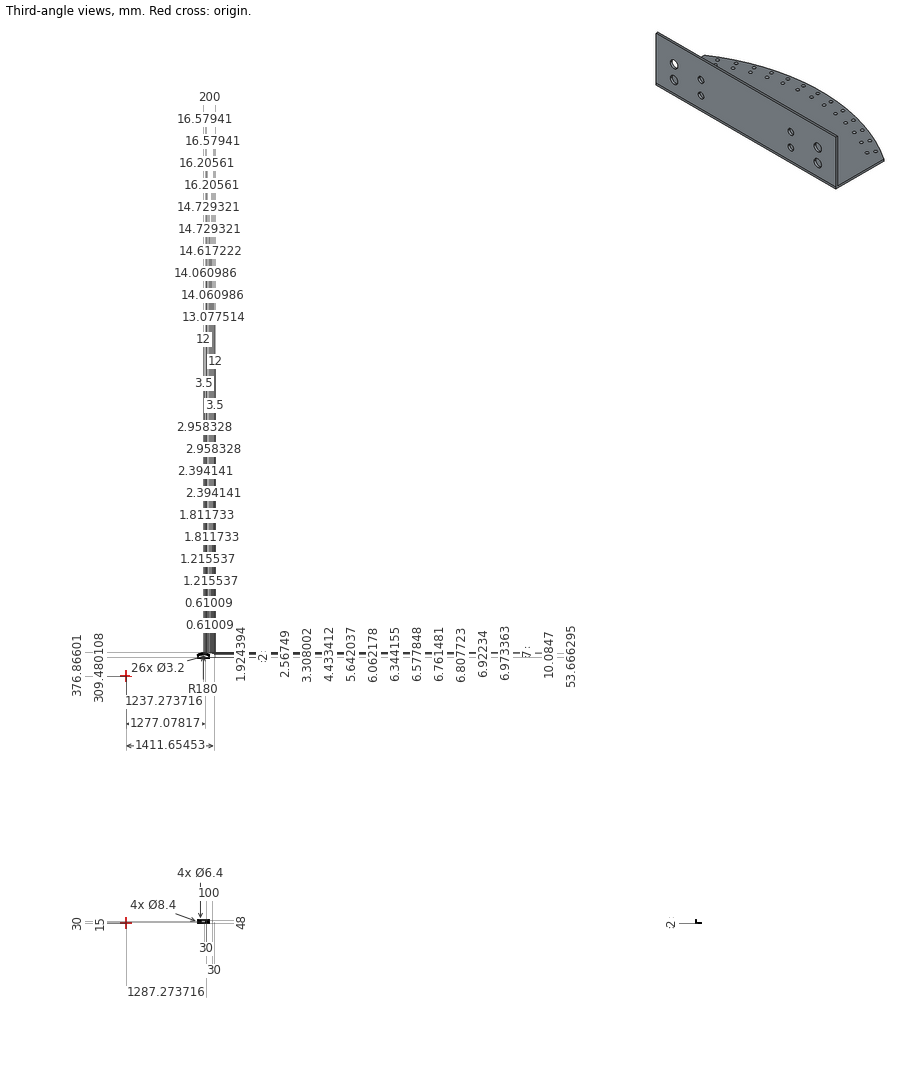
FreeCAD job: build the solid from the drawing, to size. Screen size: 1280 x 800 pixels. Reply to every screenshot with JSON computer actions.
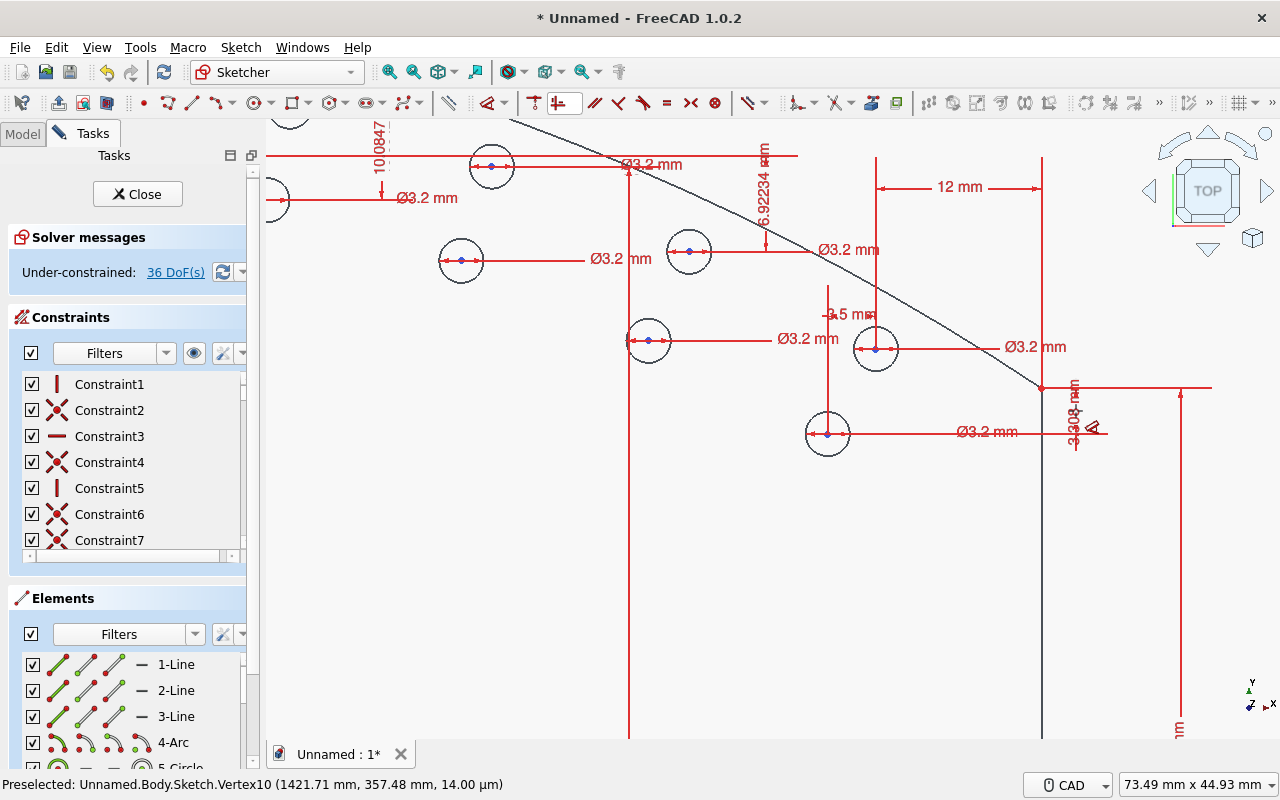
{"action": "left_click", "coordinate": [828, 434]}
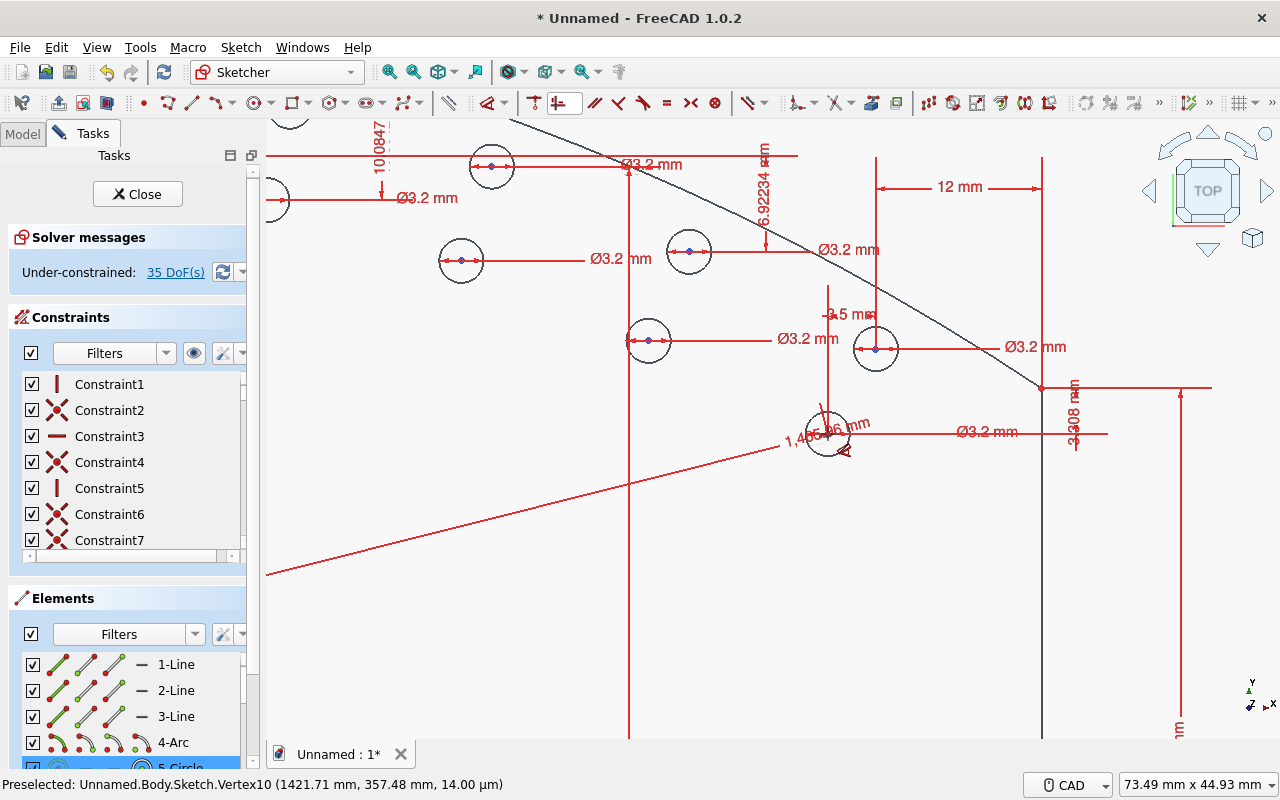
{"action": "left_click", "coordinate": [876, 349]}
{"action": "left_click", "coordinate": [910, 392]}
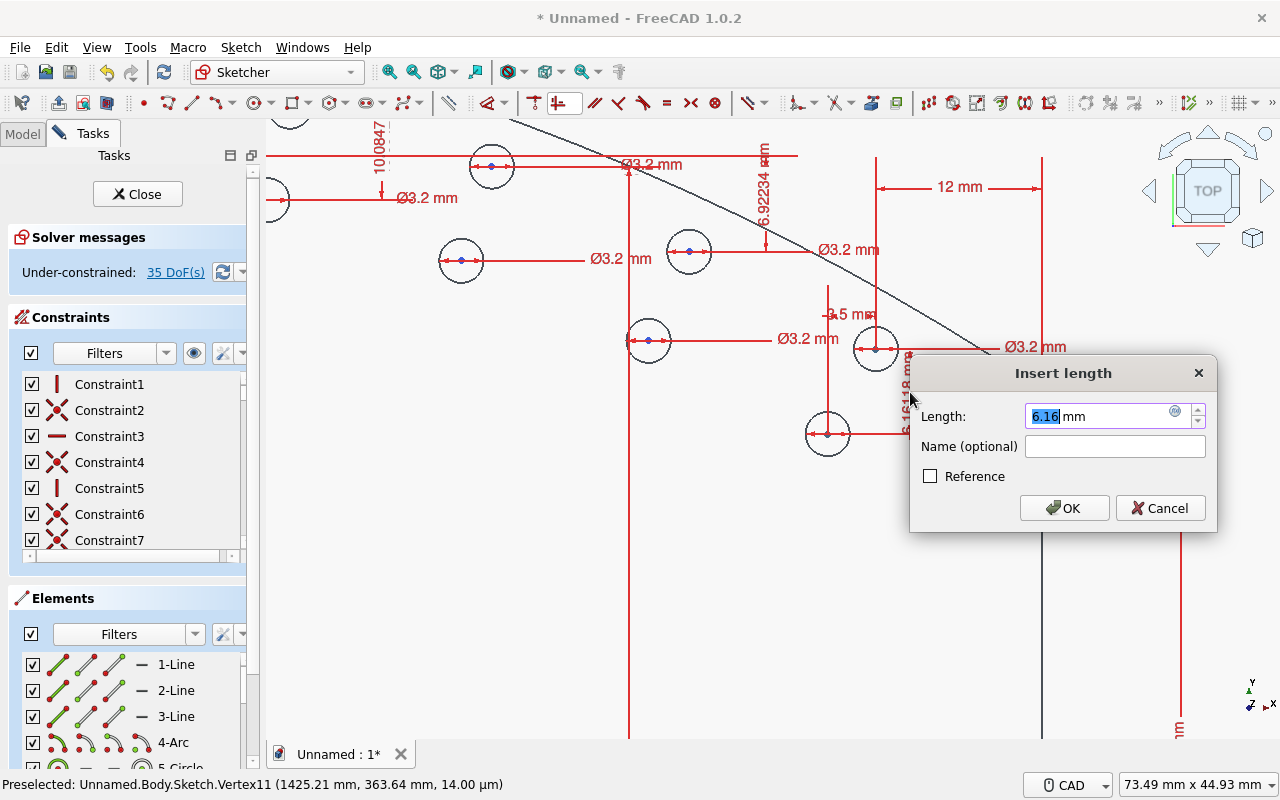
{"action": "type", "text": "6.062178"}
{"action": "key", "text": "Return"}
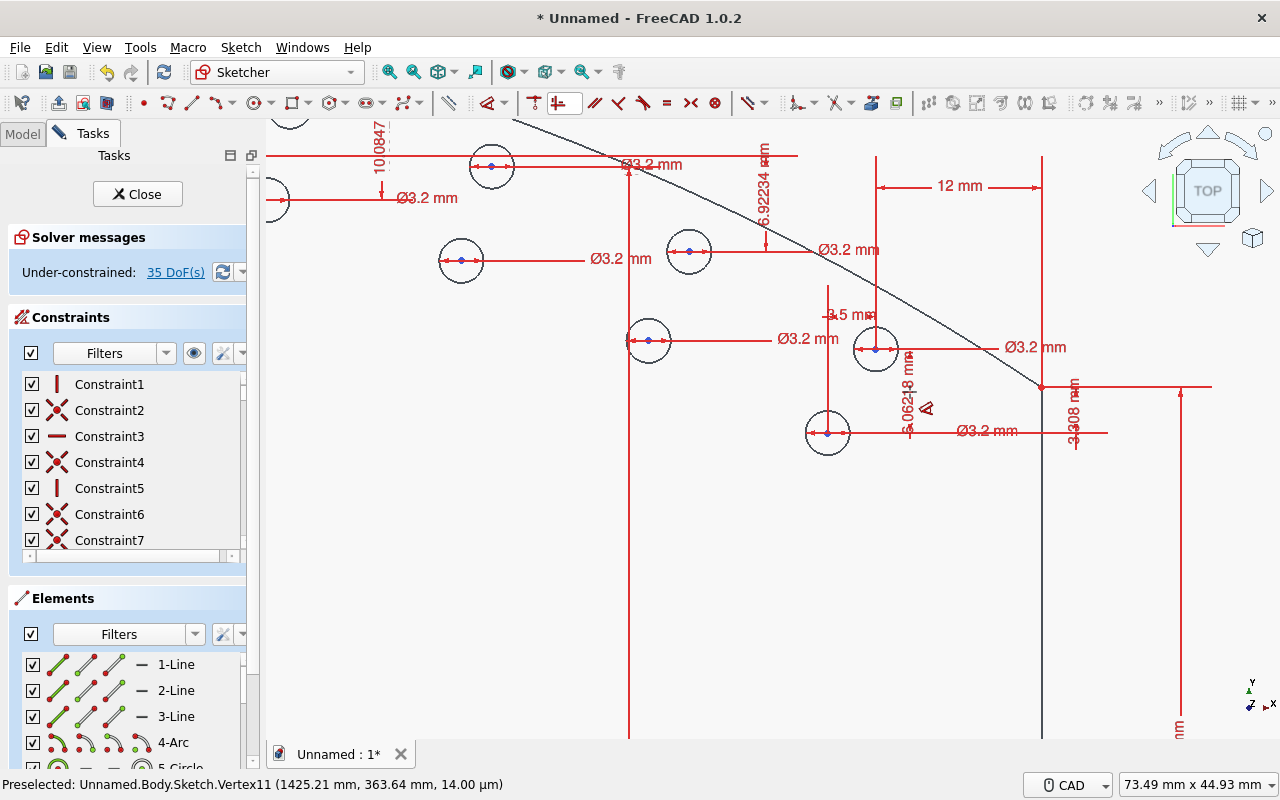
{"action": "left_click", "coordinate": [828, 433]}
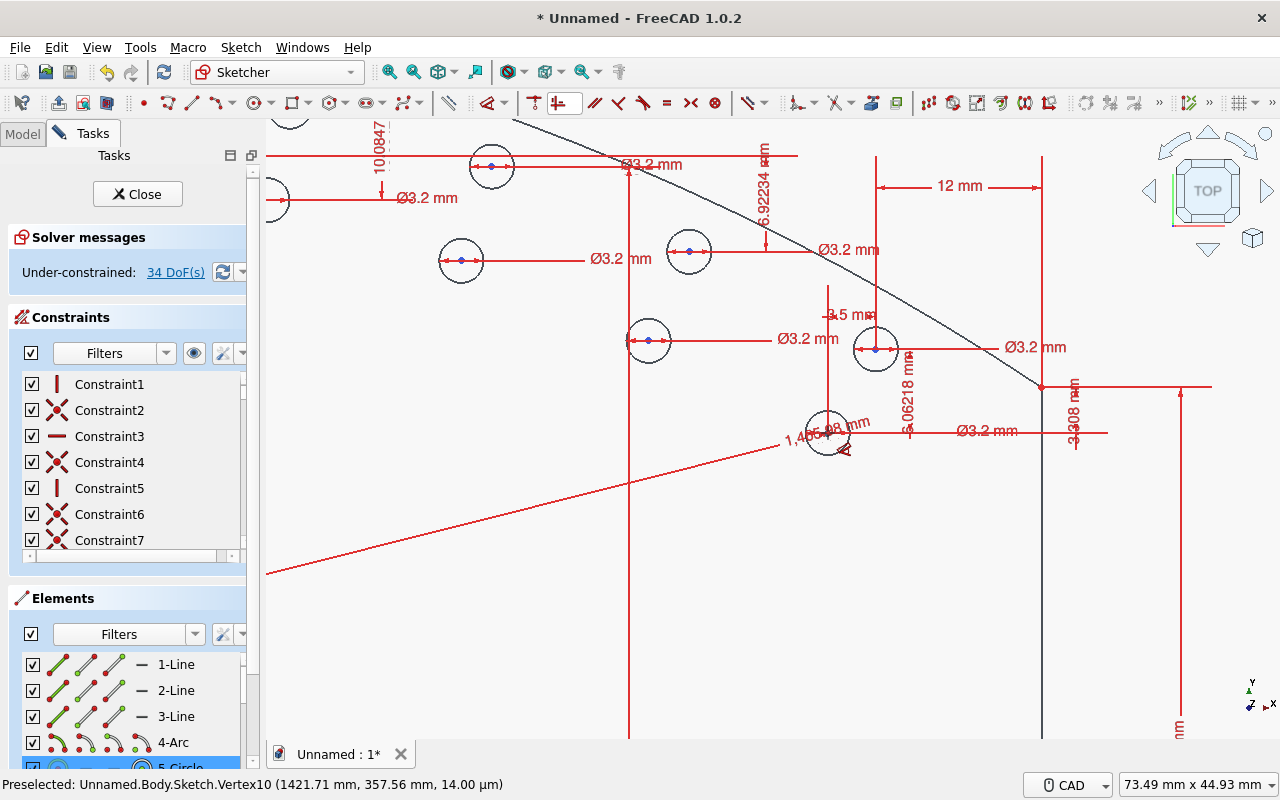
{"action": "left_click", "coordinate": [649, 341]}
{"action": "left_click", "coordinate": [862, 419]}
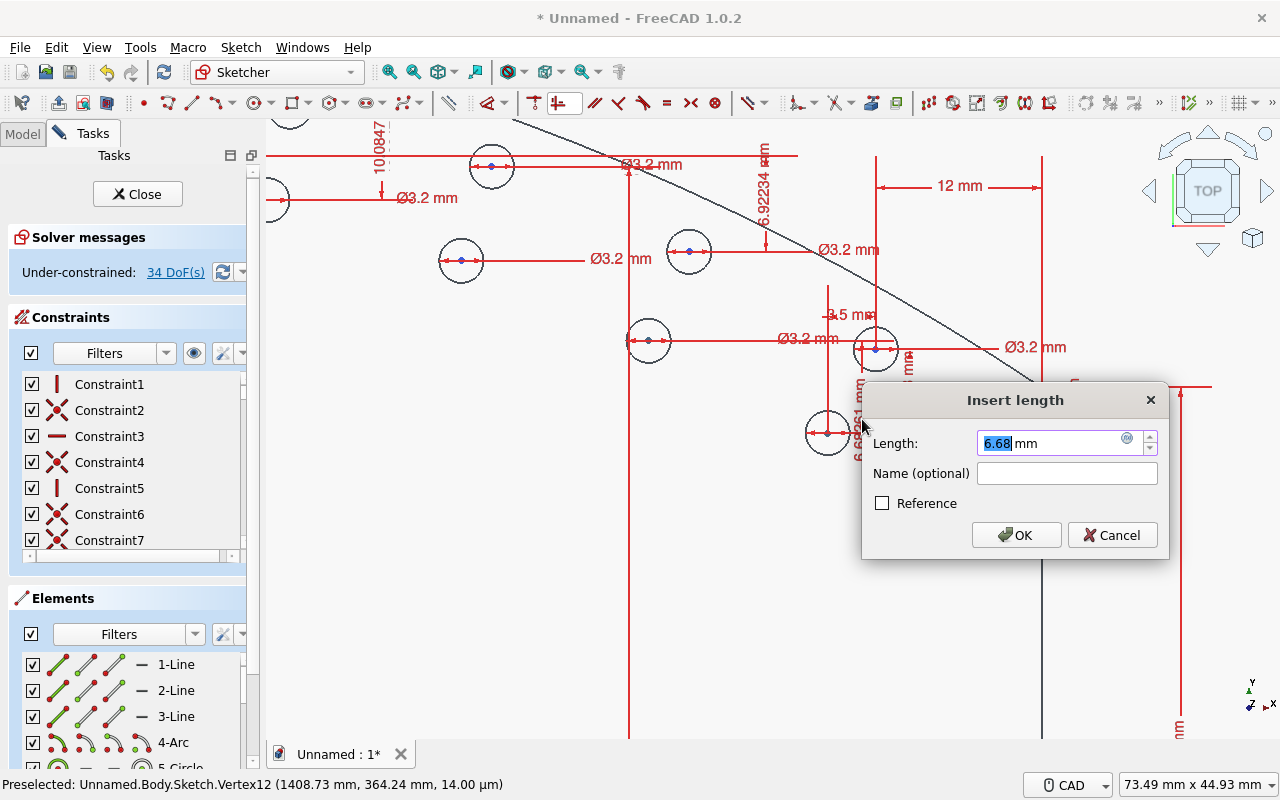
{"action": "type", "text": "6.807723"}
{"action": "key", "text": "Return"}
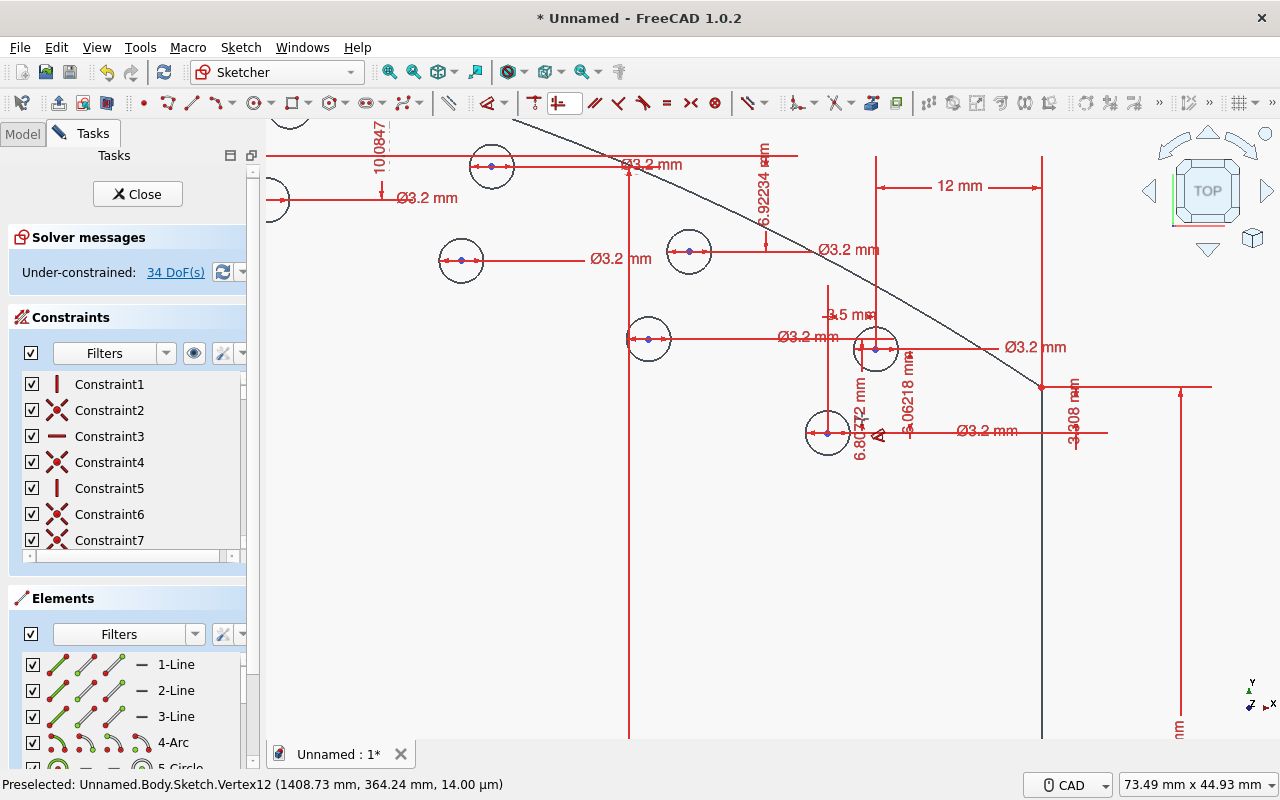
{"action": "left_click", "coordinate": [649, 339]}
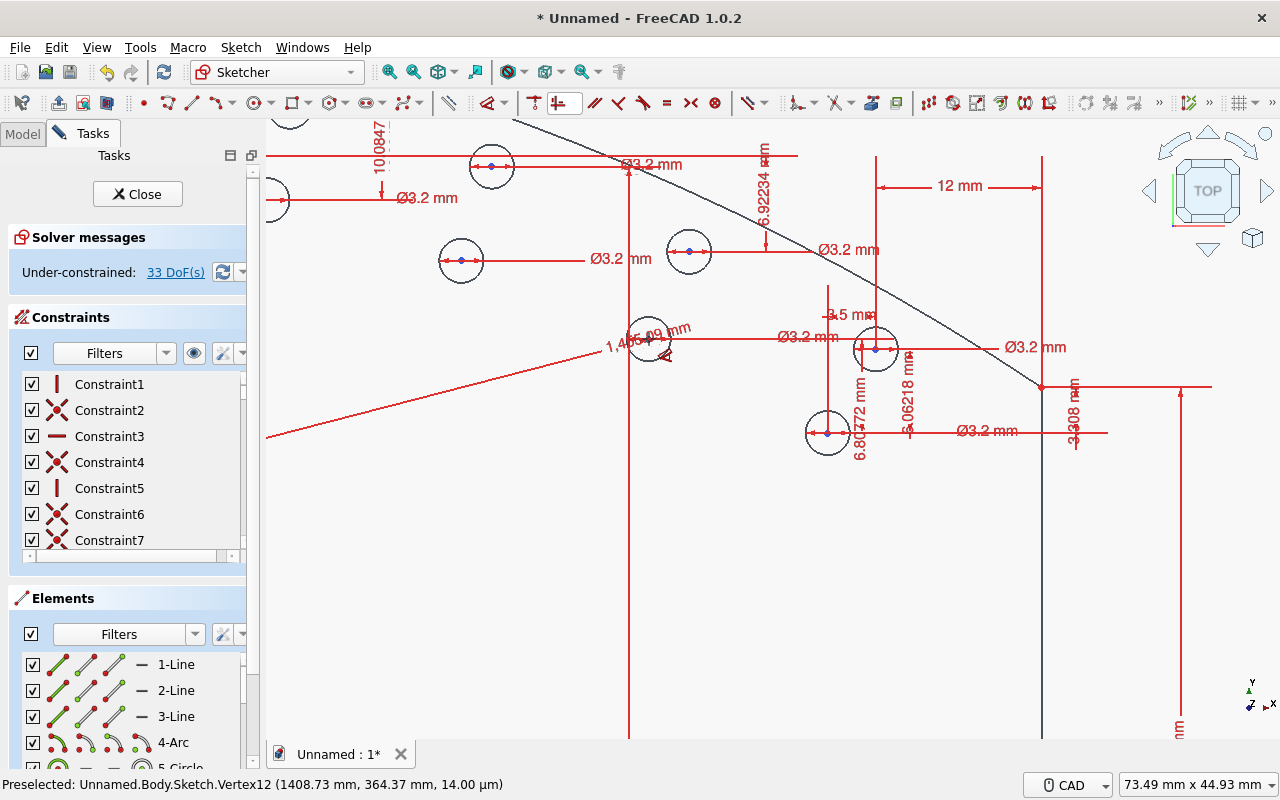
{"action": "left_click", "coordinate": [689, 252]}
{"action": "left_click", "coordinate": [669, 218]}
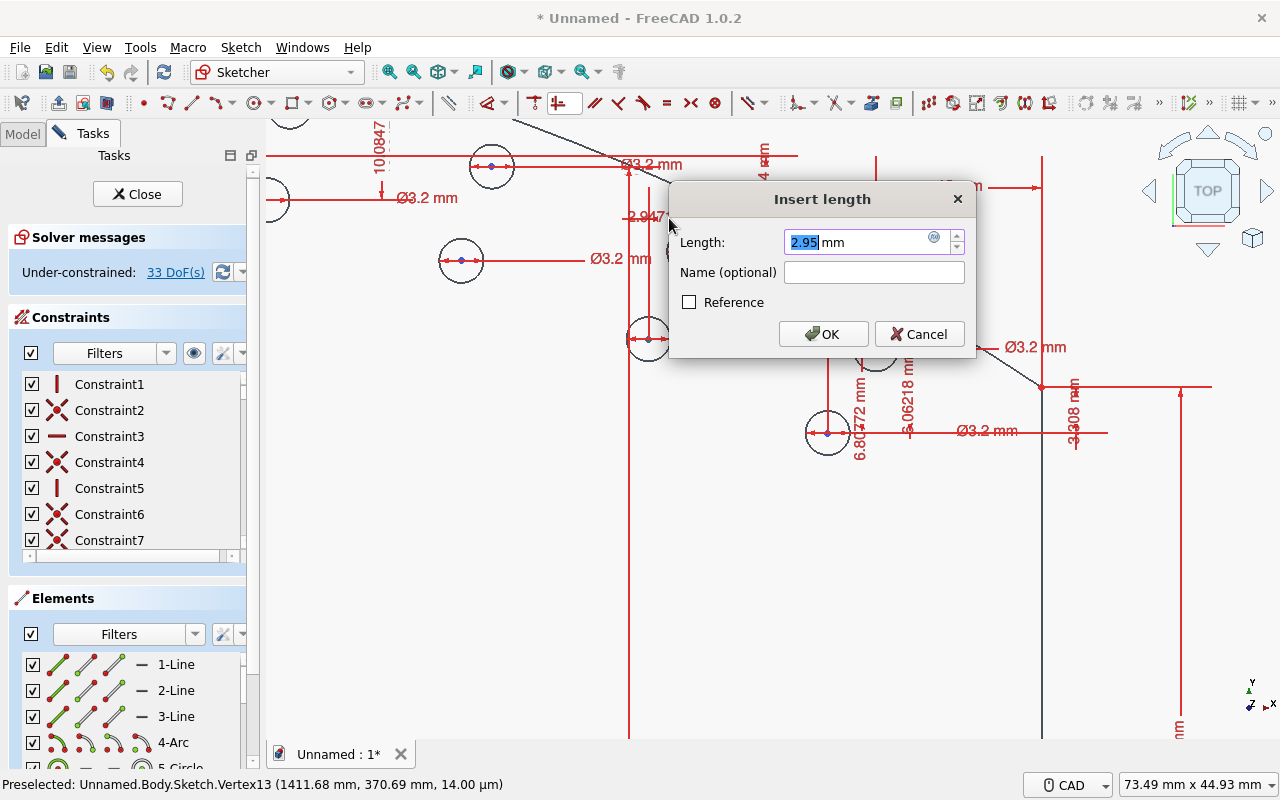
{"action": "type", "text": "2.958328"}
{"action": "key", "text": "Return"}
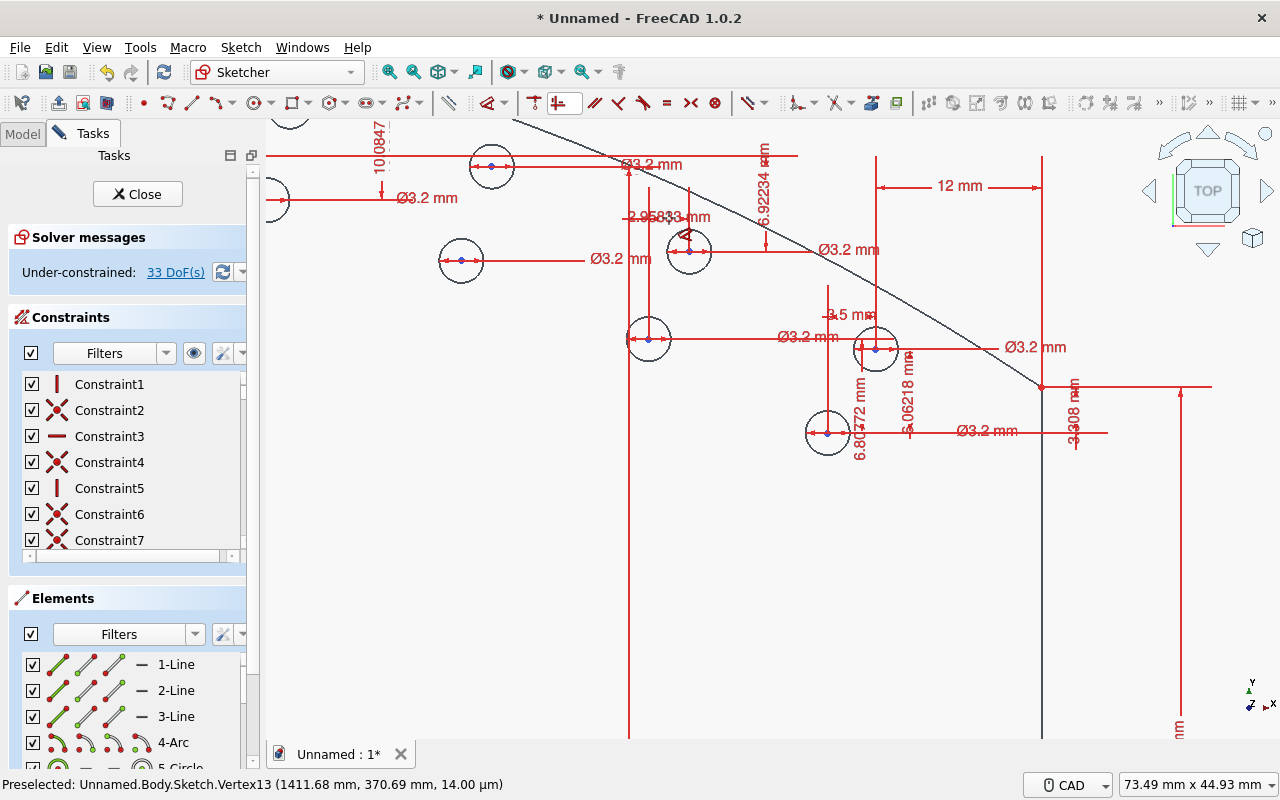
{"action": "left_click", "coordinate": [649, 339]}